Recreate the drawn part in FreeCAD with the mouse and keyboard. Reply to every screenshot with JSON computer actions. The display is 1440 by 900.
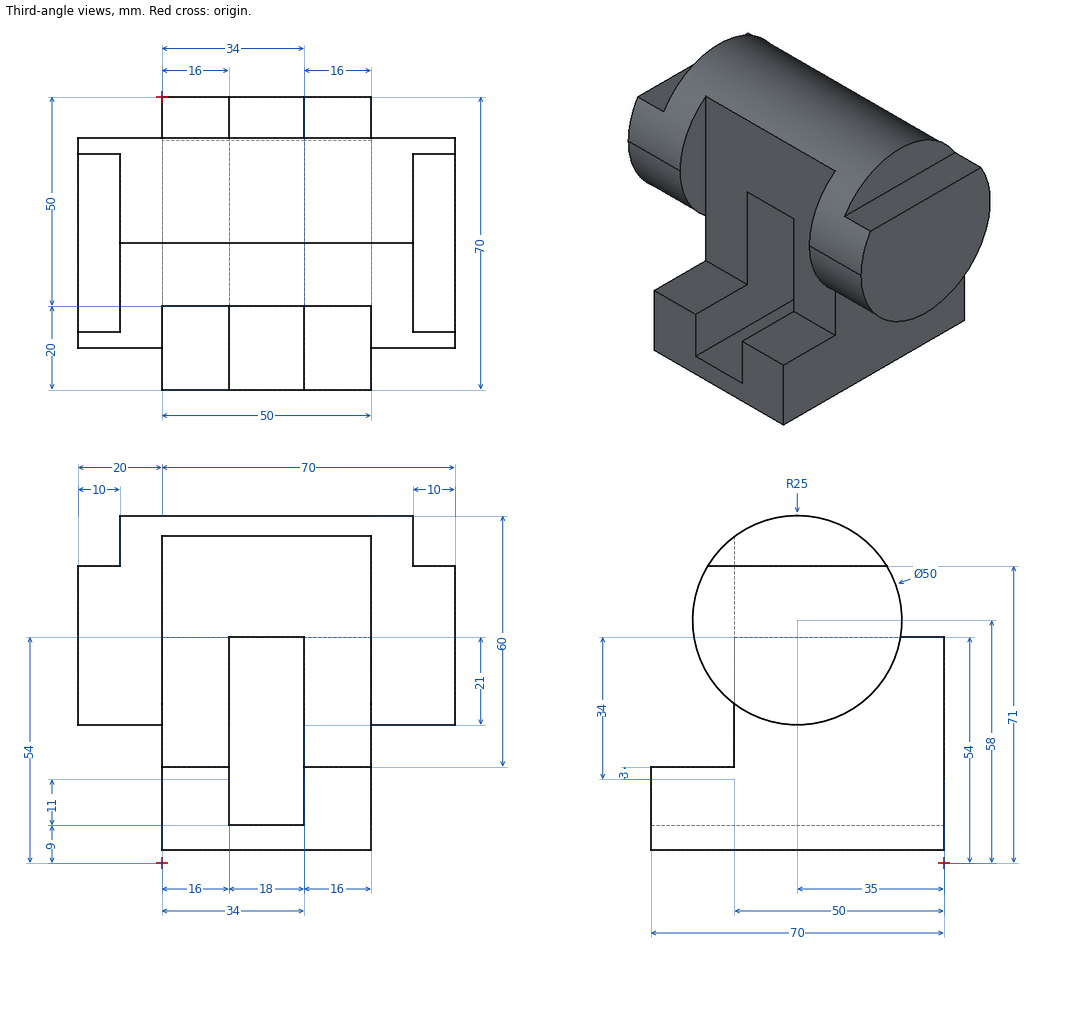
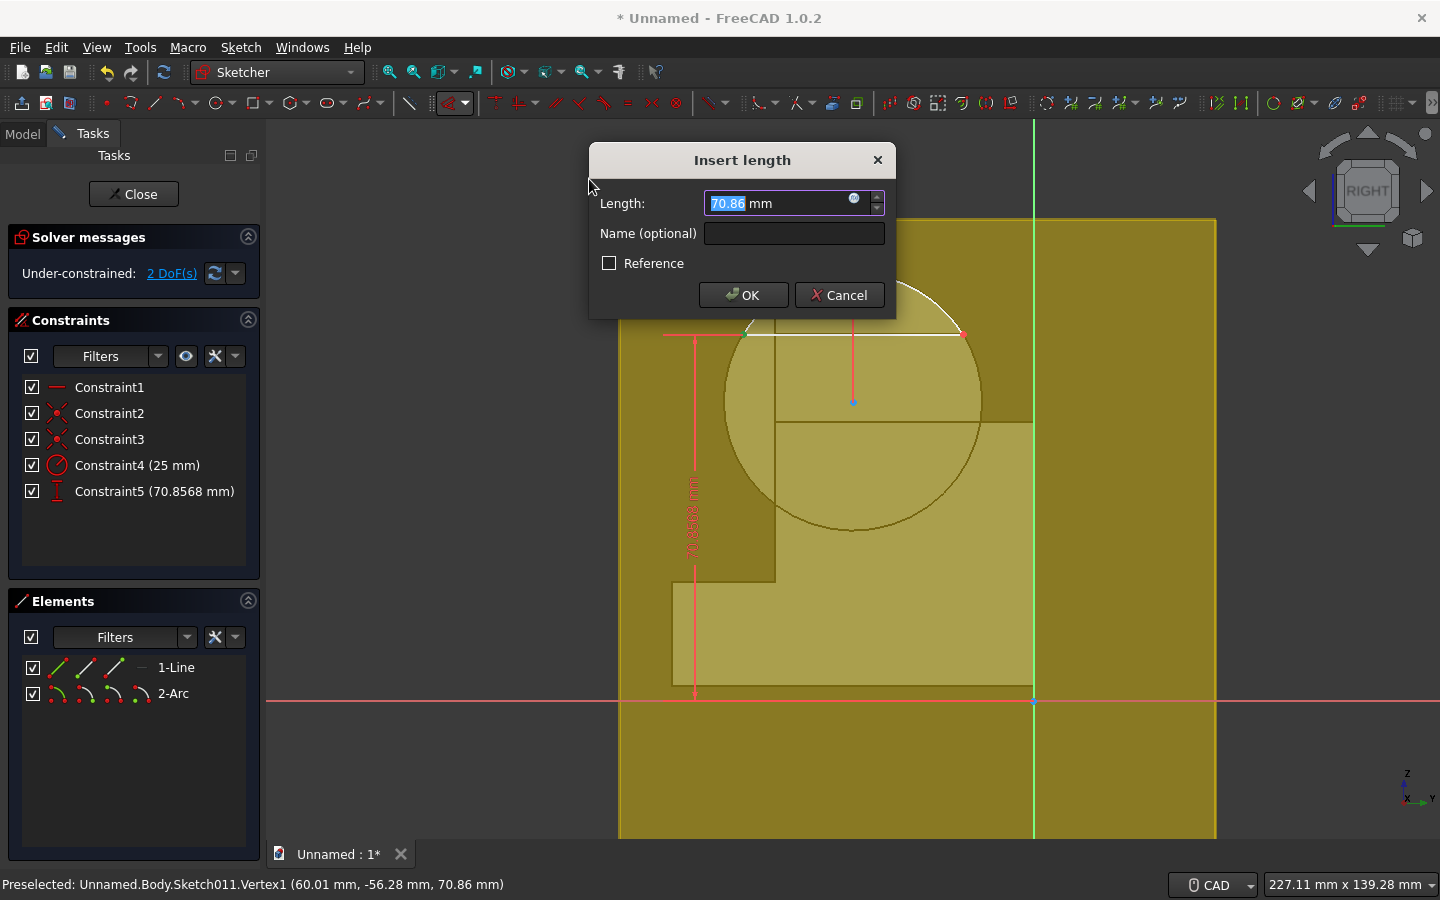
{"action": "type", "text": "71"}
{"action": "key", "text": "Return"}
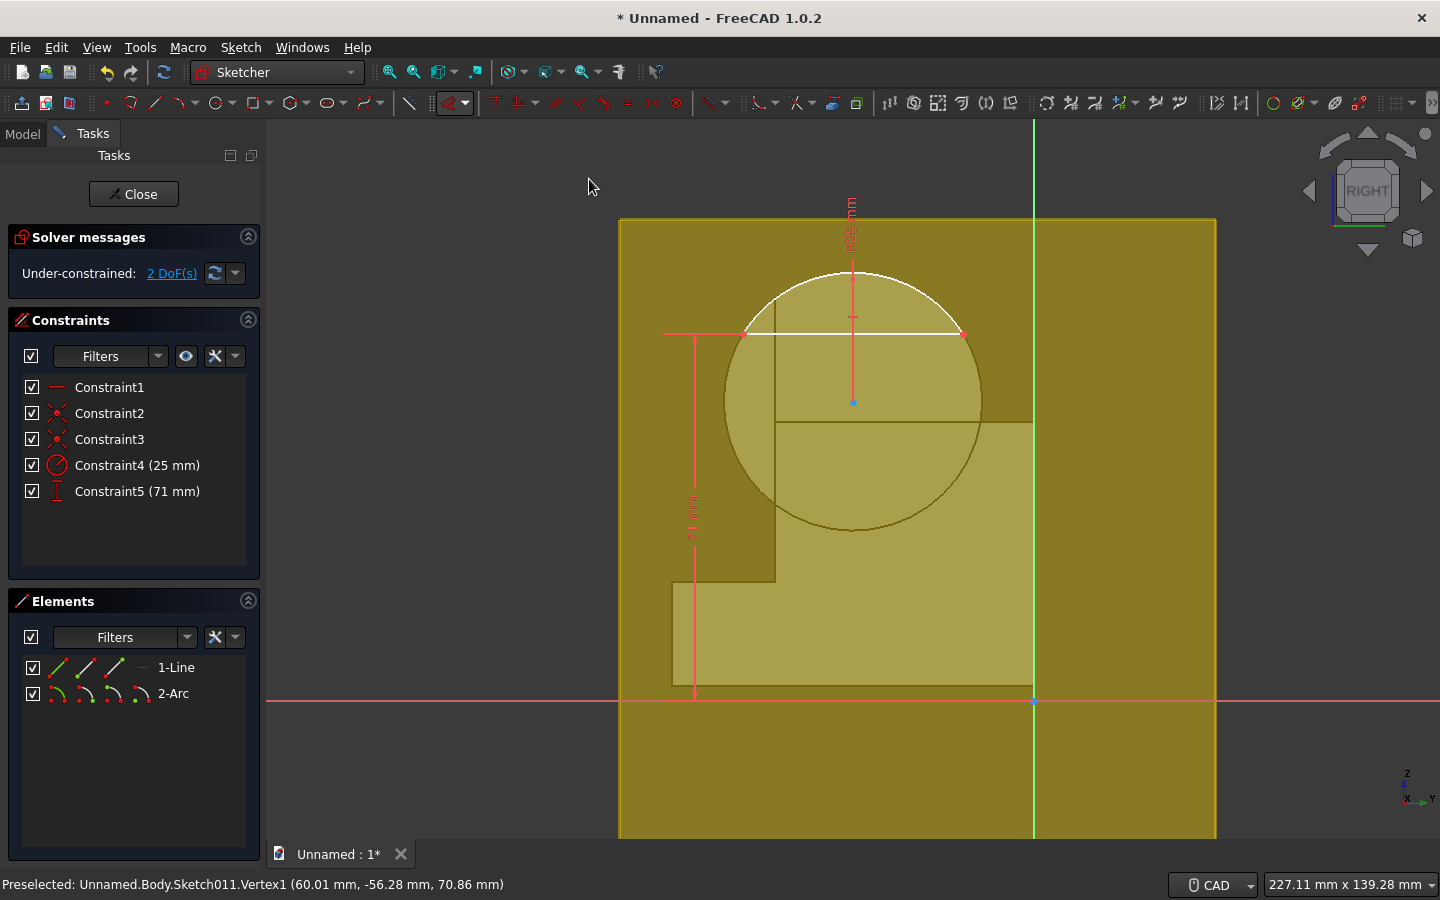
{"action": "left_click", "coordinate": [853, 402]}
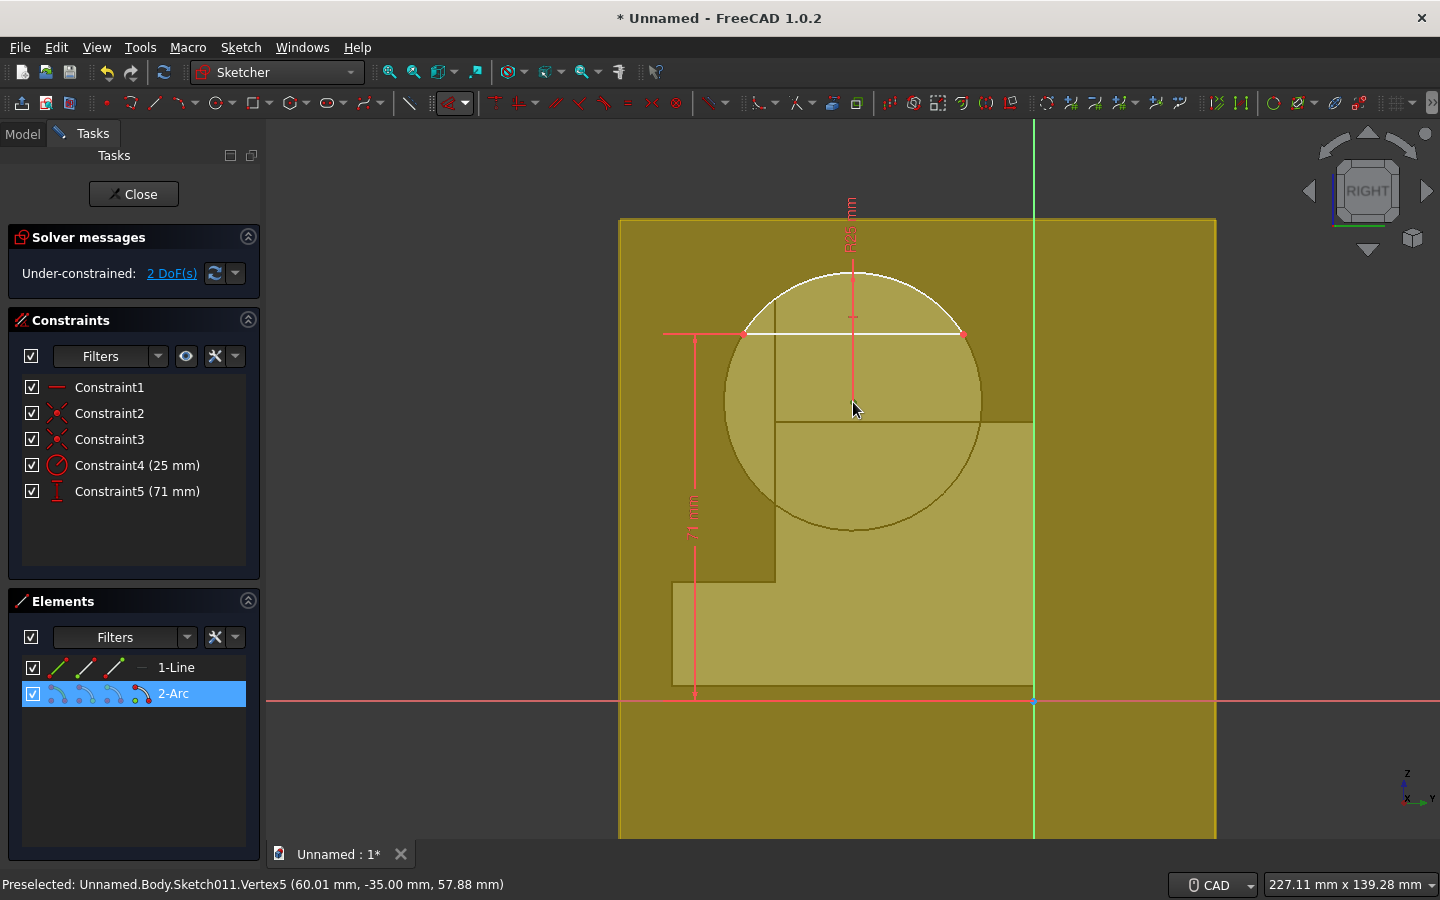
{"action": "key", "text": "l"}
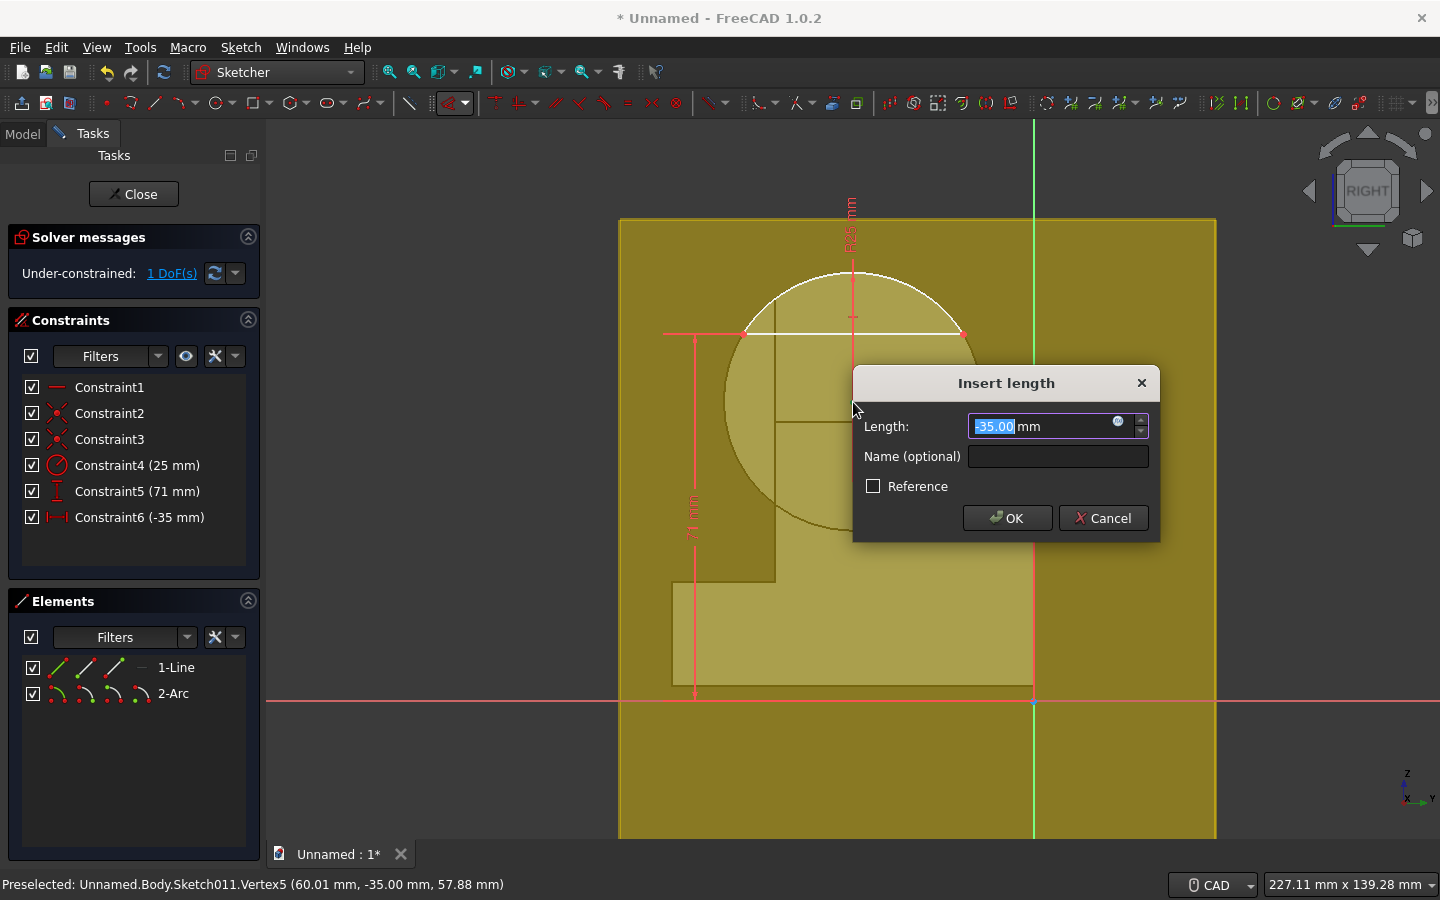
{"action": "type", "text": "-35"}
{"action": "key", "text": "Return"}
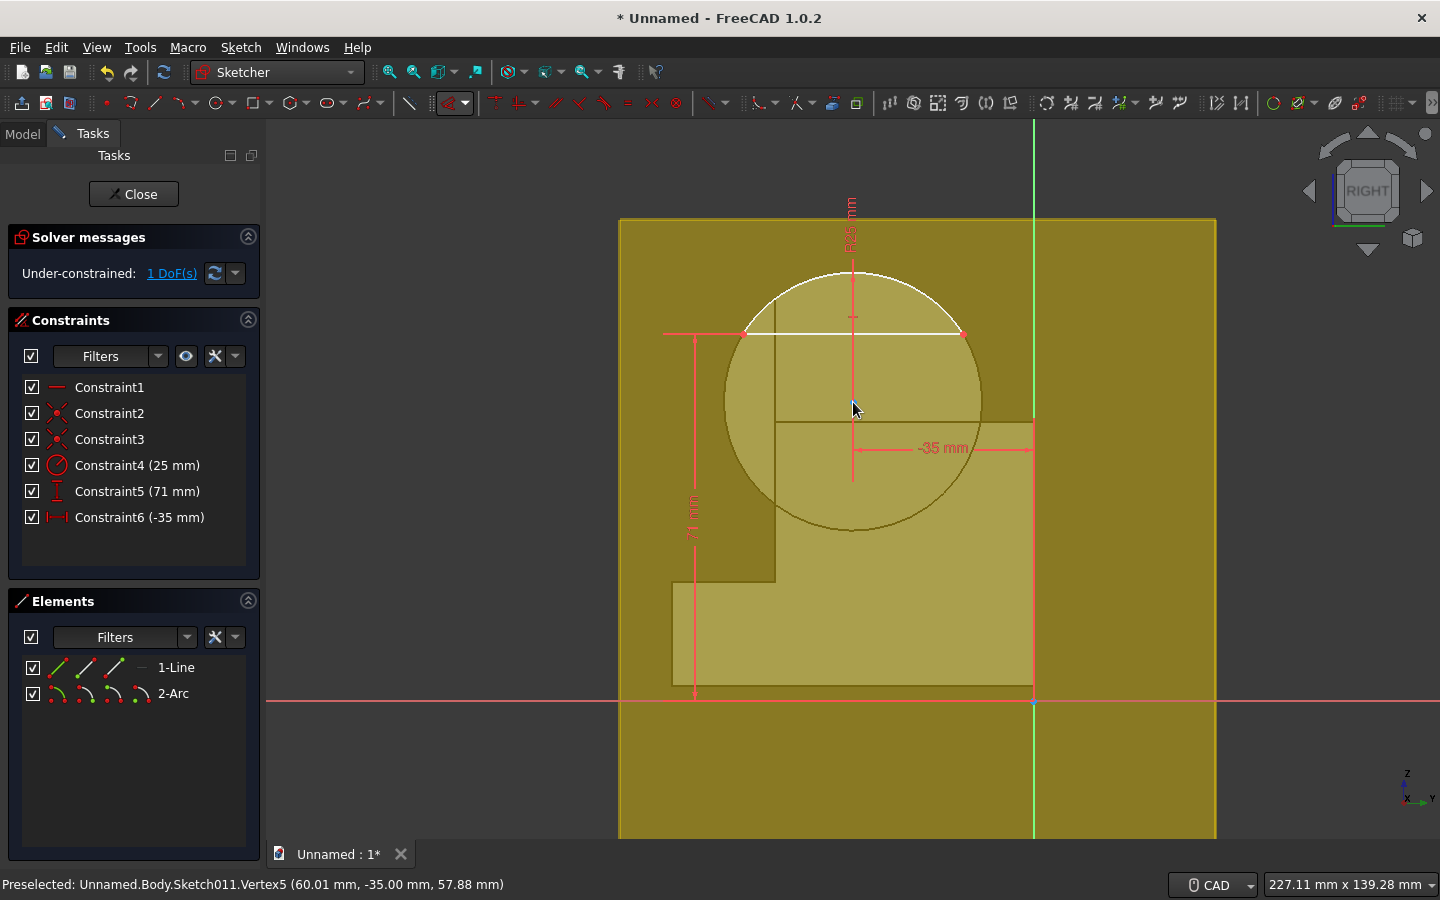
{"action": "left_click", "coordinate": [853, 402]}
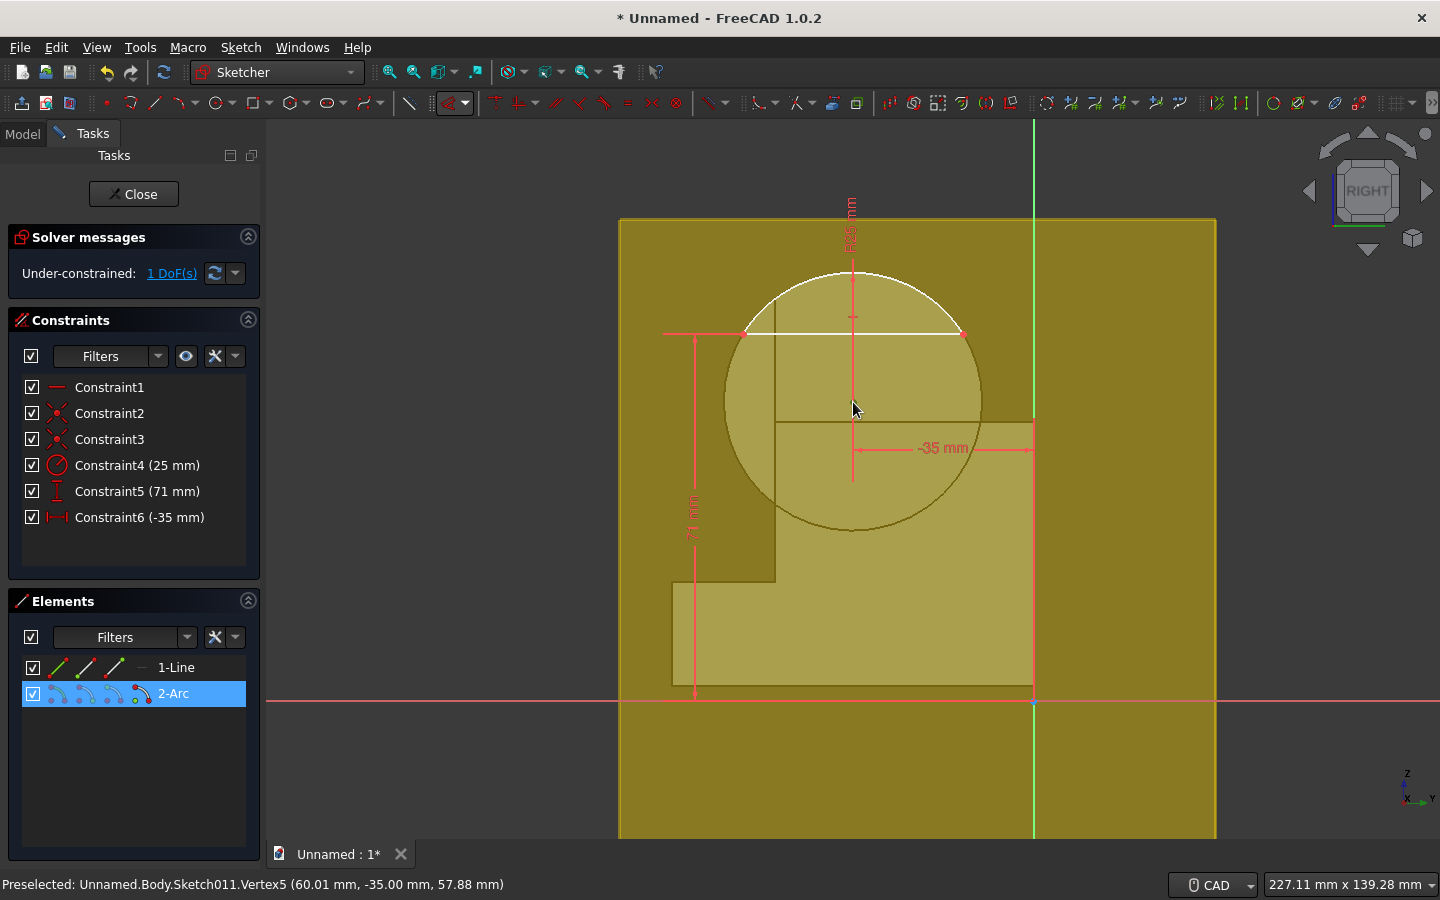
{"action": "key", "text": "i"}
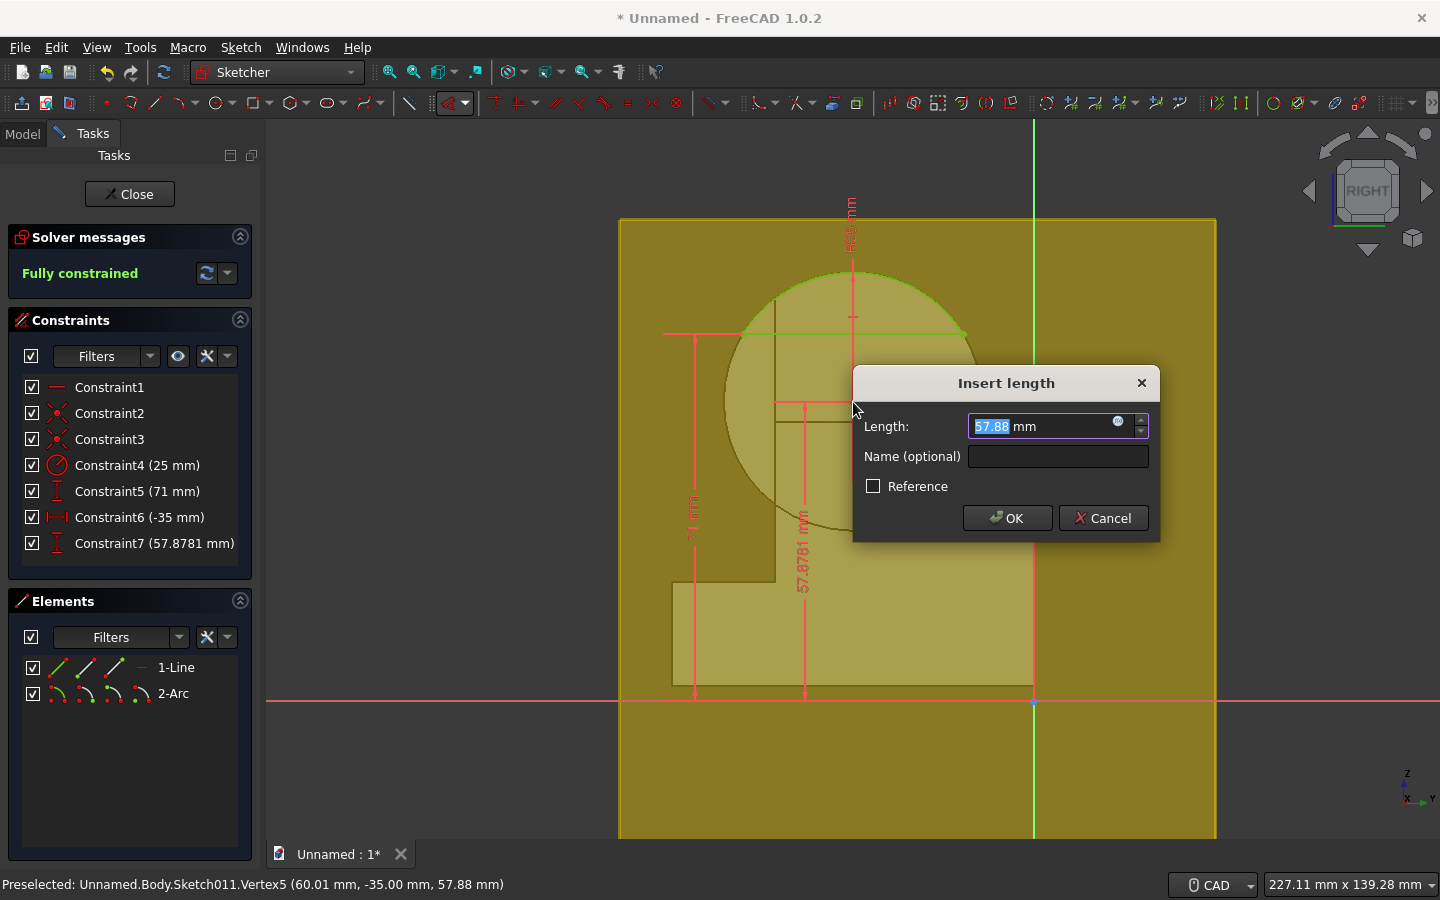
{"action": "type", "text": "58"}
{"action": "key", "text": "Return"}